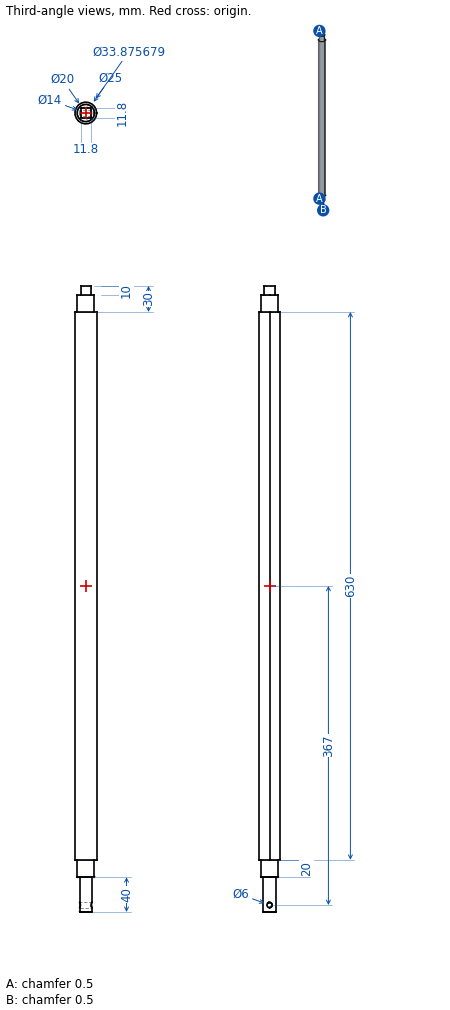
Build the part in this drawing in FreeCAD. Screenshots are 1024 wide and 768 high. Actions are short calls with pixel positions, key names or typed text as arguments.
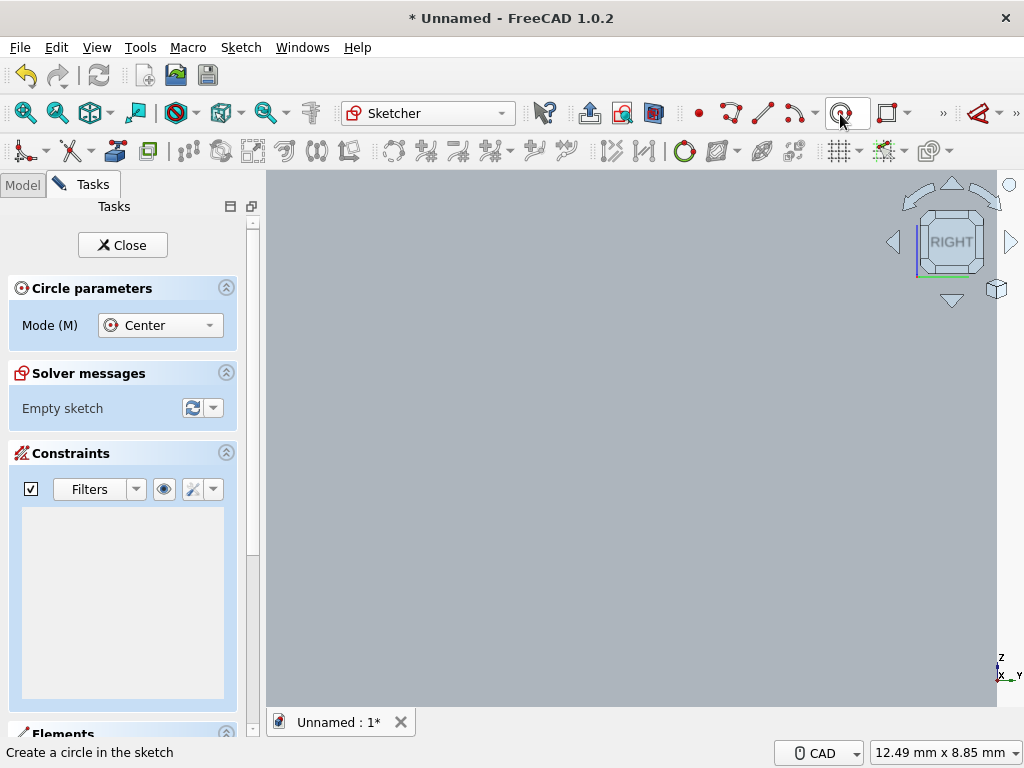
click(576, 438)
move(704, 309)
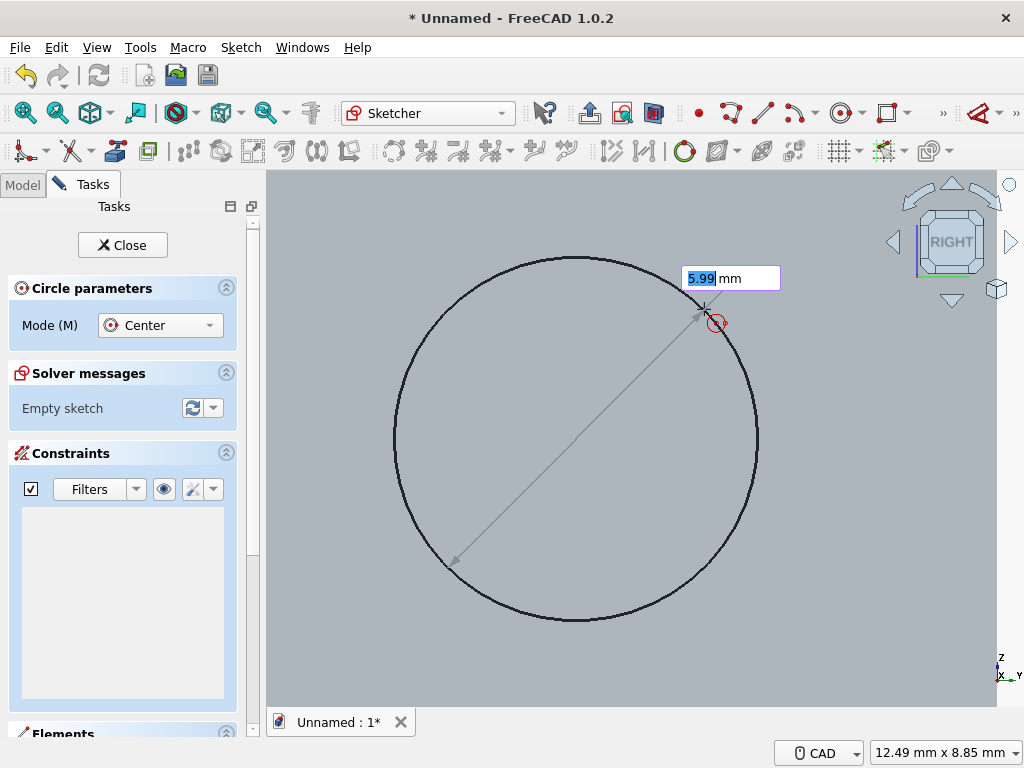
text(6)
key(Return)
key(Escape)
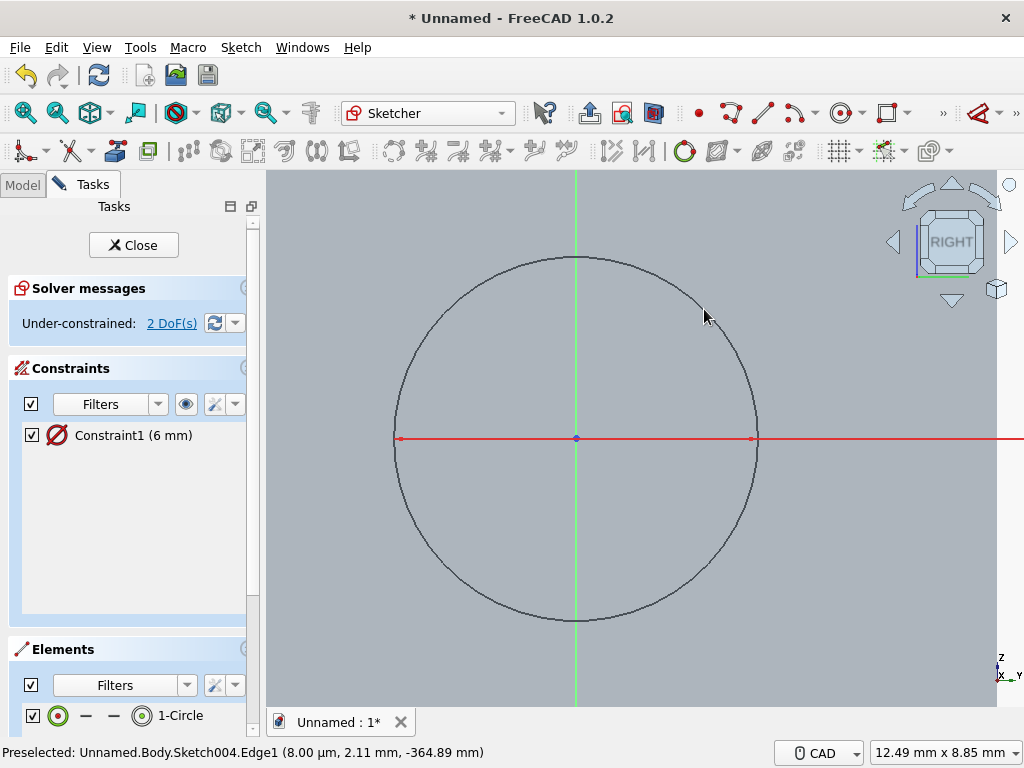
click(576, 439)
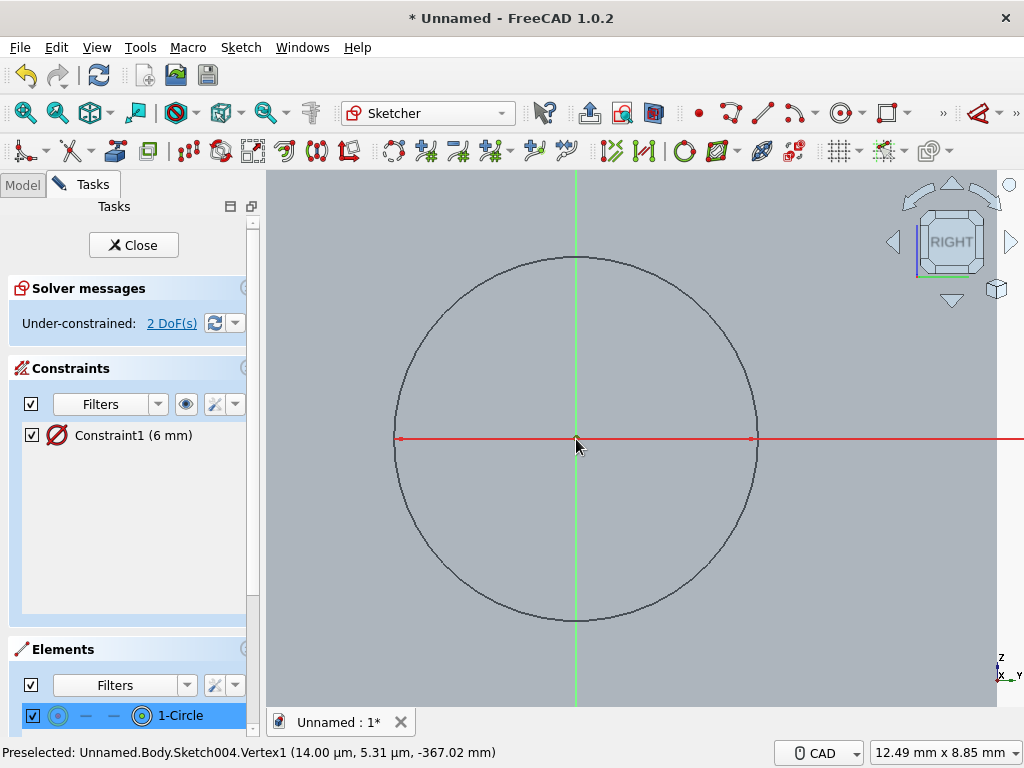
click(576, 576)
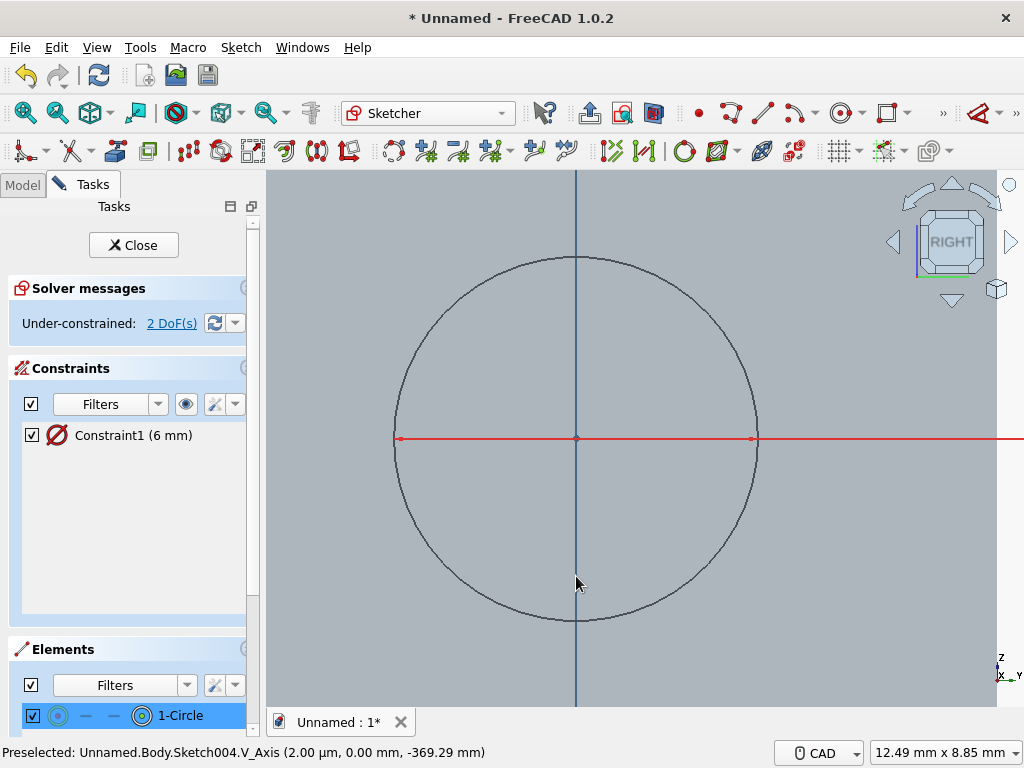
key(c)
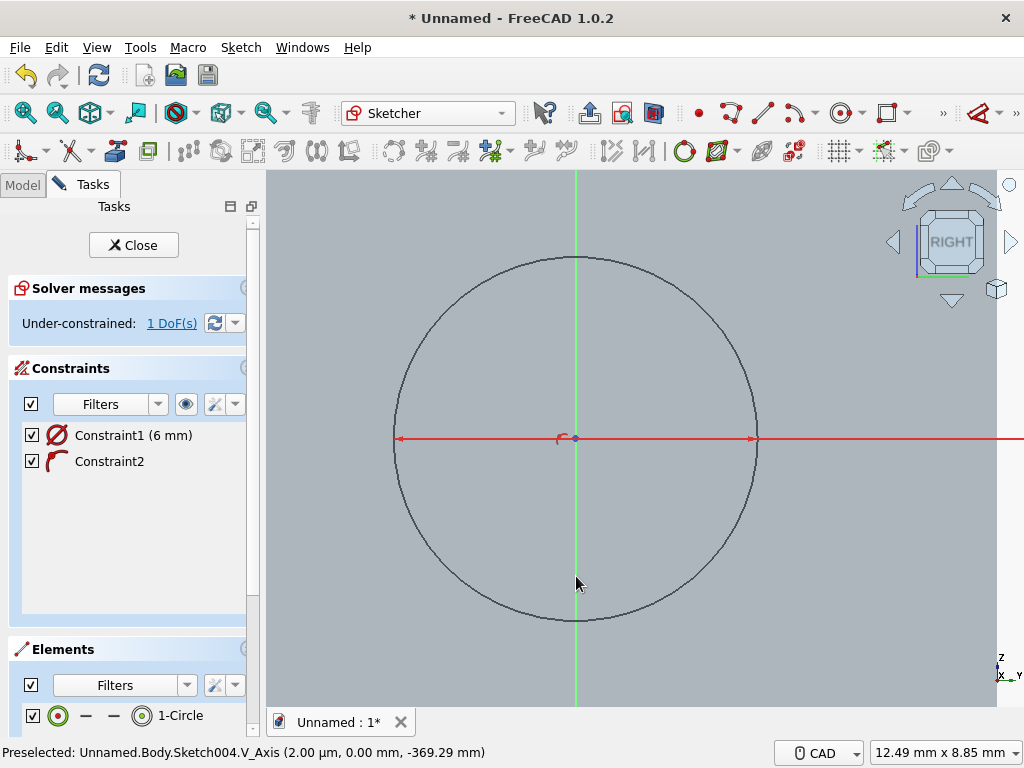
click(978, 114)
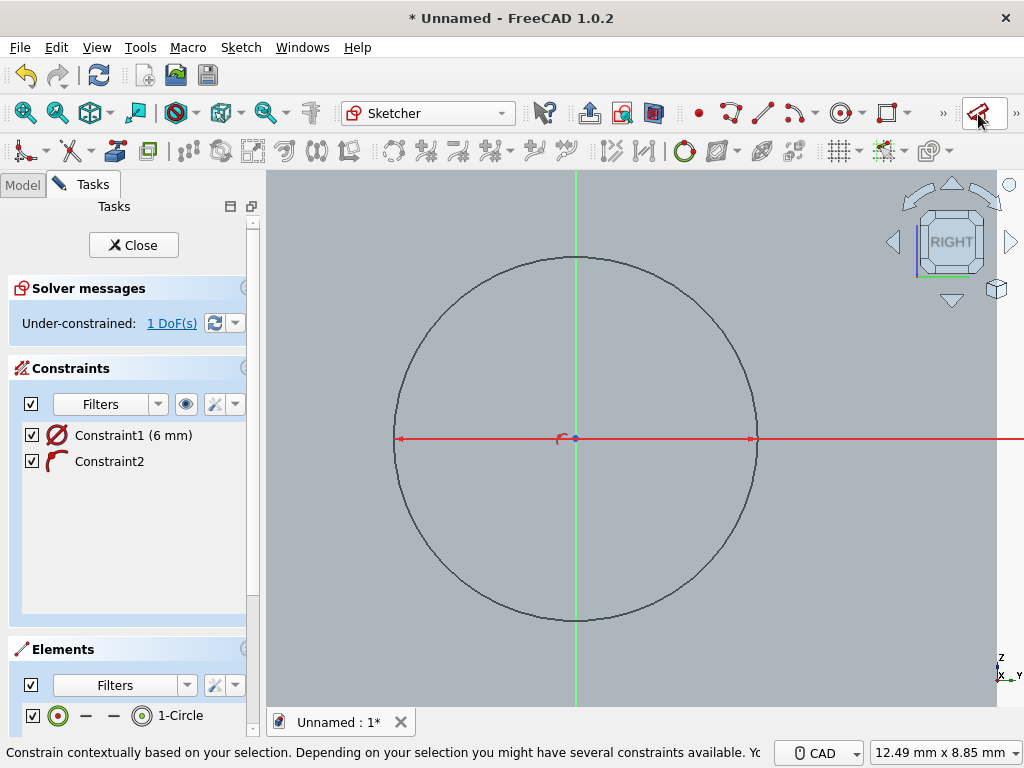
click(576, 439)
click(610, 318)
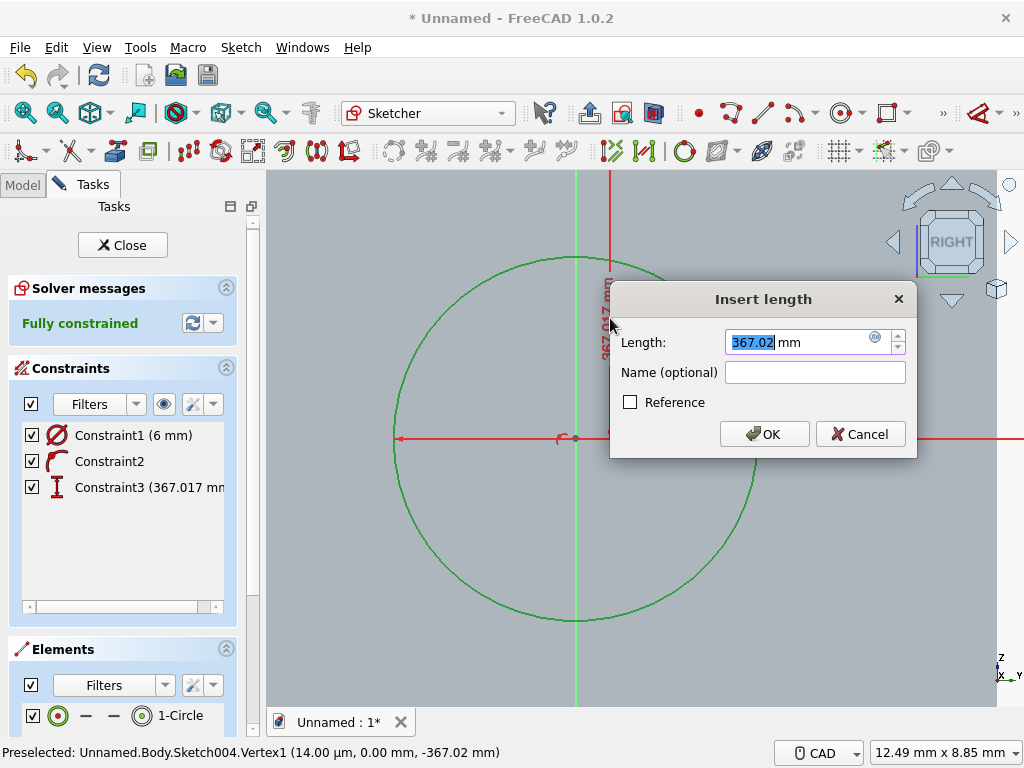
text(367)
key(Return)
key(Escape)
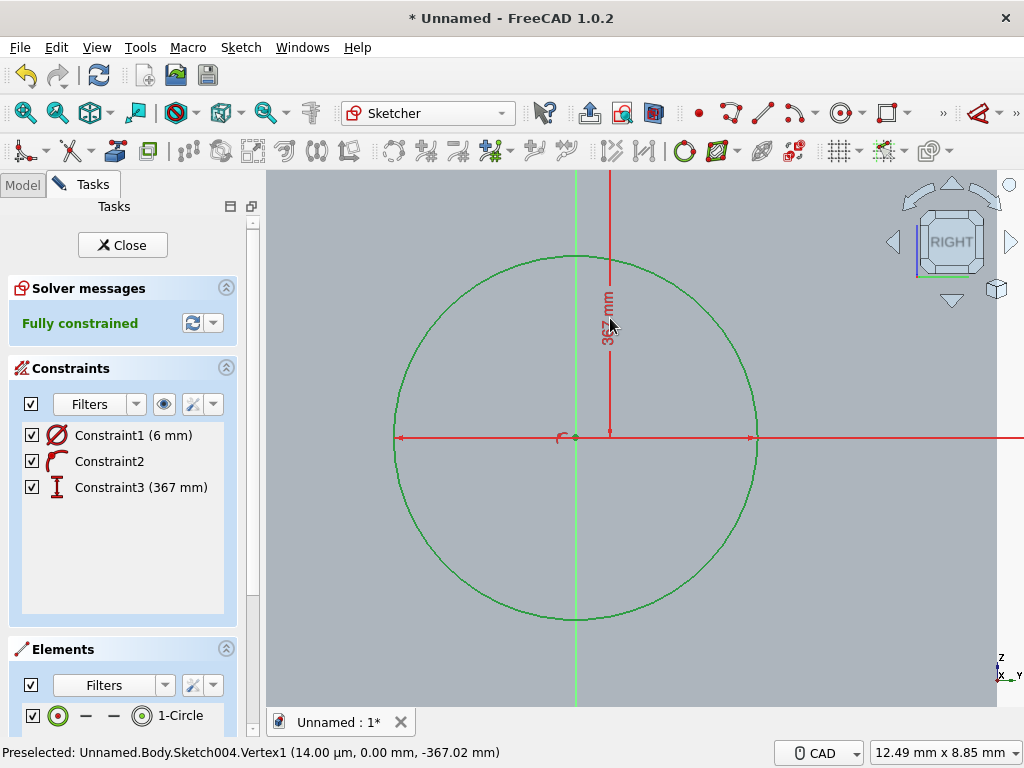
click(123, 245)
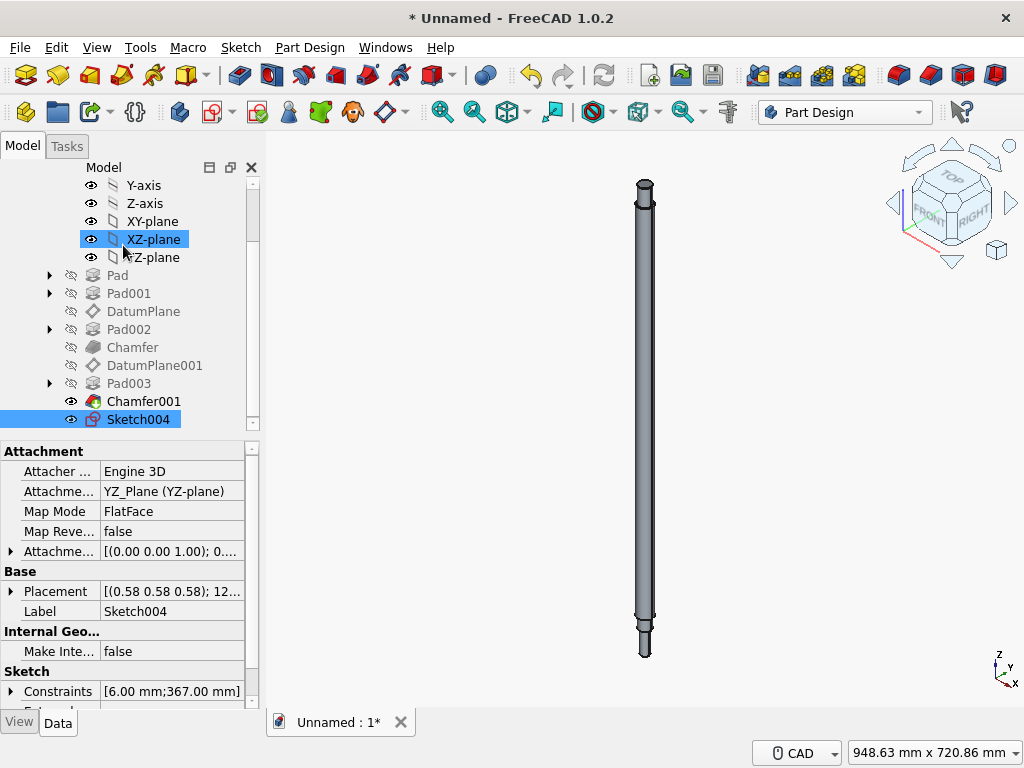
click(240, 76)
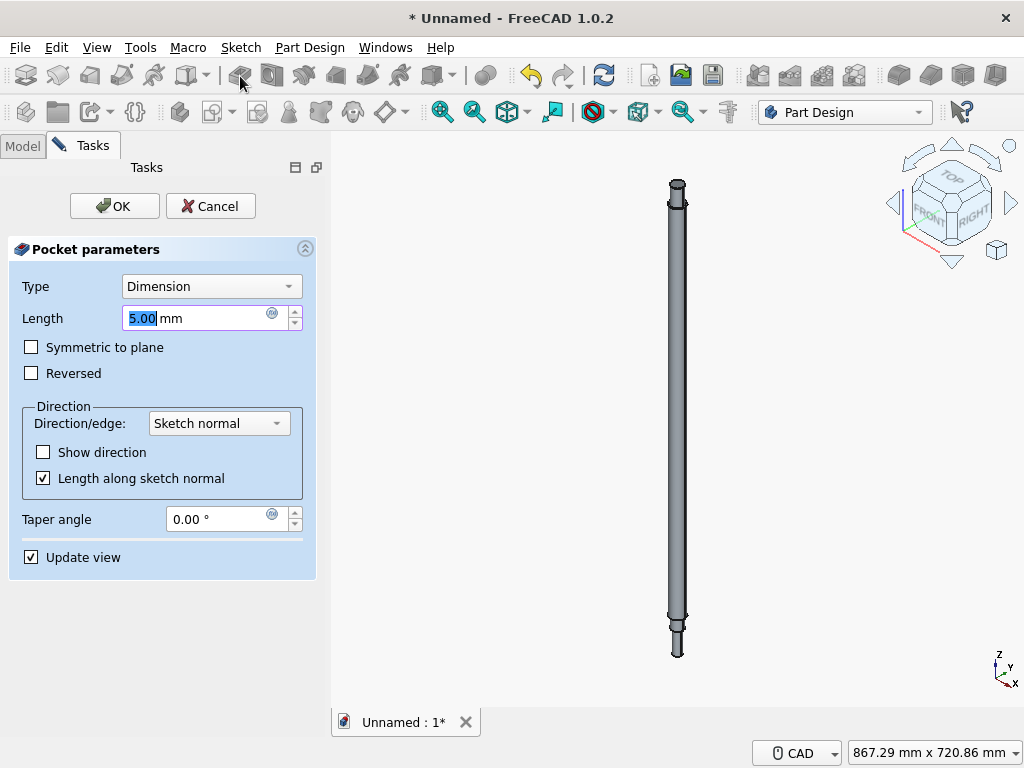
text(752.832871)
key(Tab)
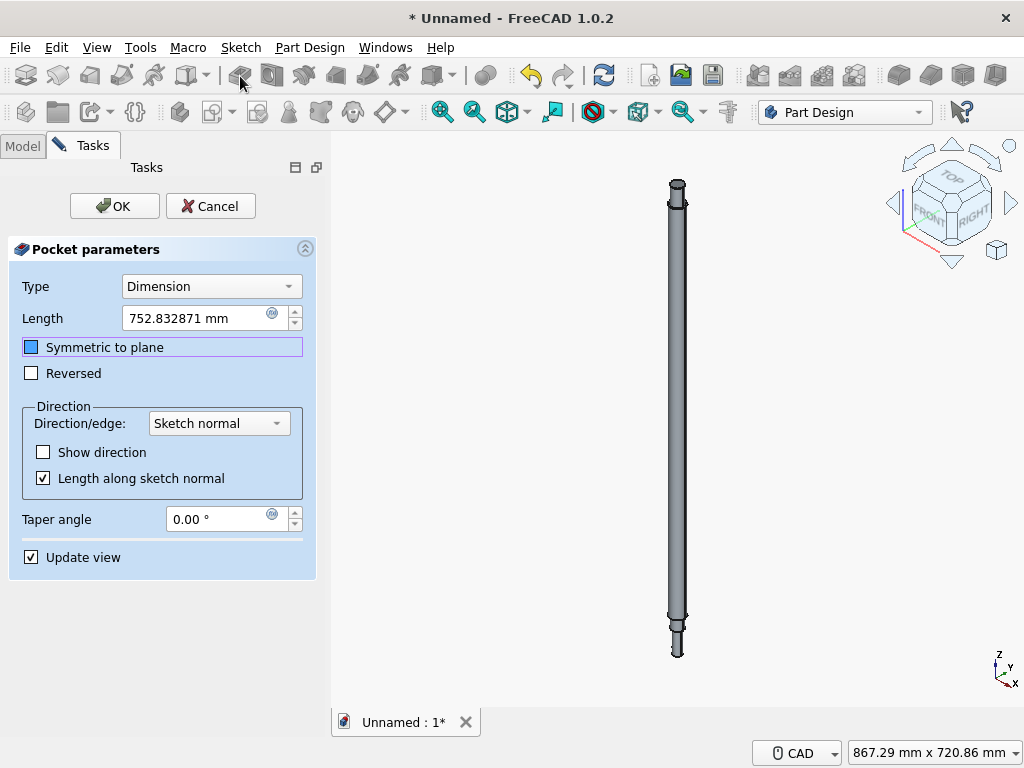
click(30, 347)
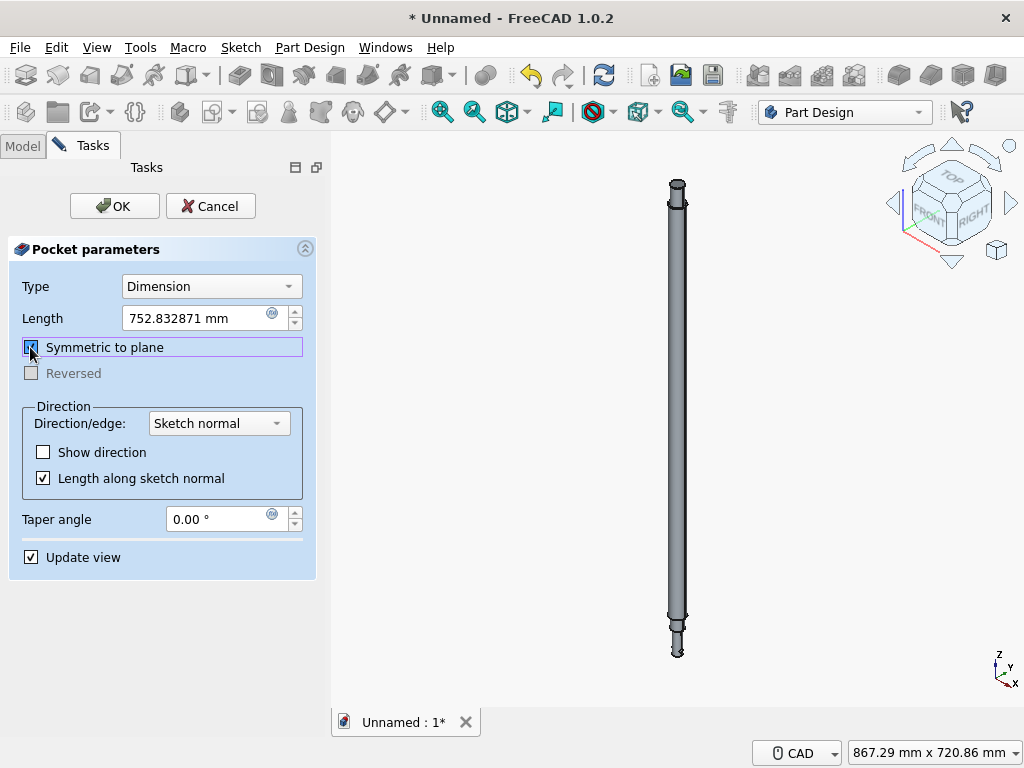
click(115, 206)